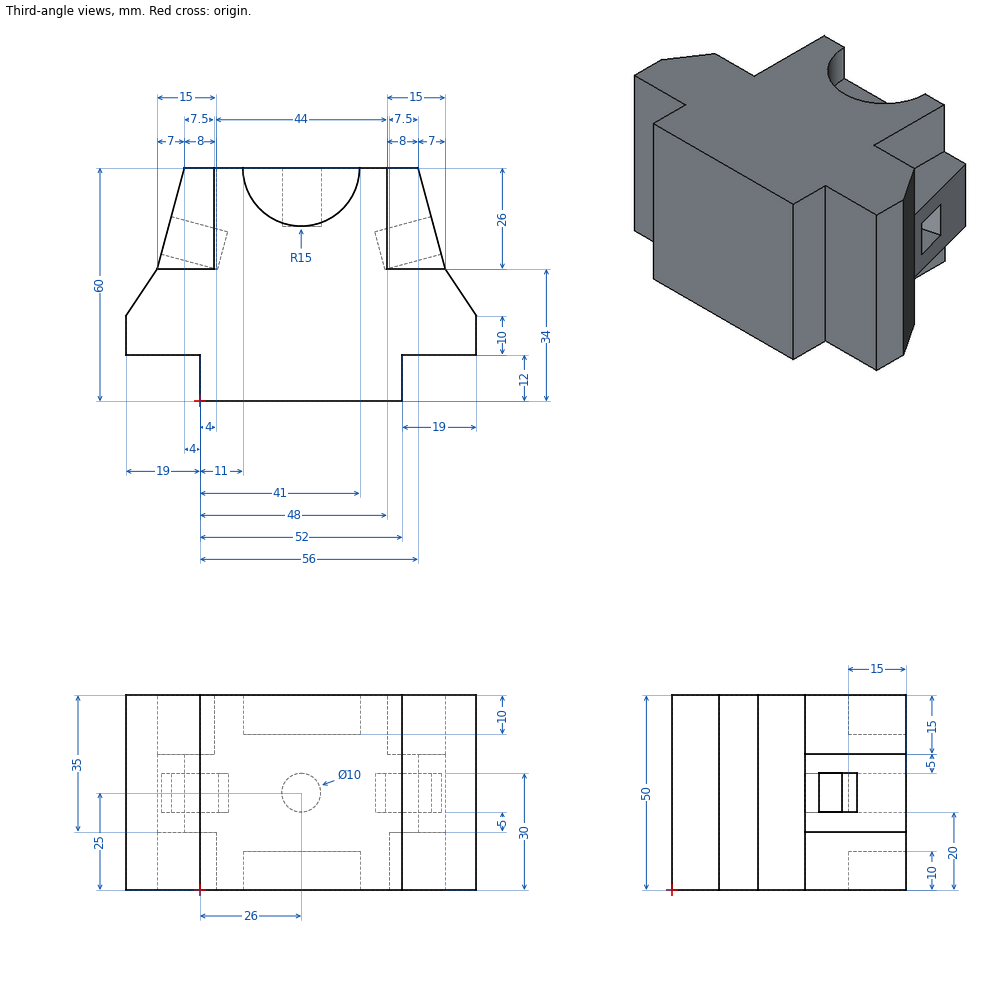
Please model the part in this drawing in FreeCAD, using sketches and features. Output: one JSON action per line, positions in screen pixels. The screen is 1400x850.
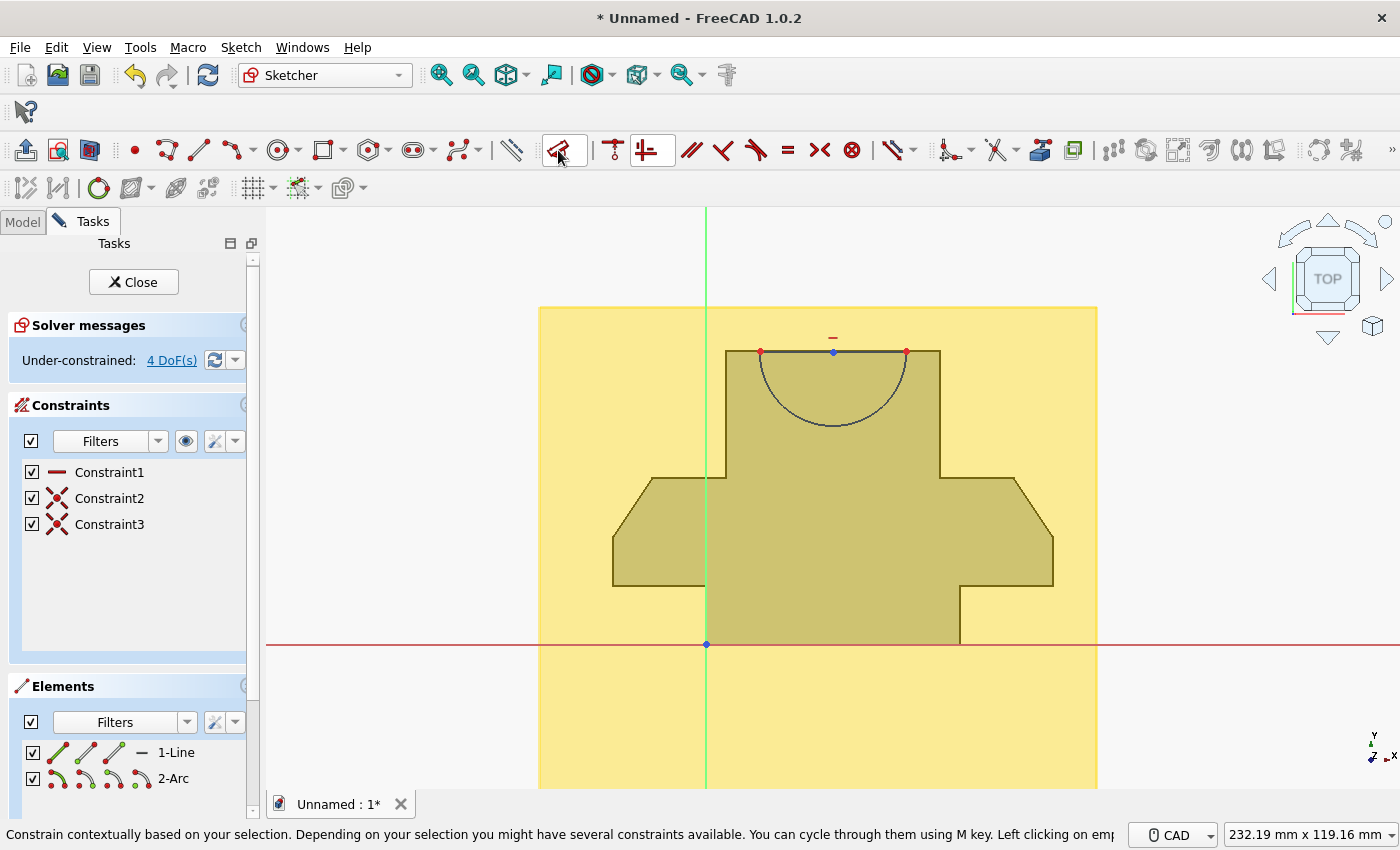
{"action": "left_click", "coordinate": [790, 412]}
{"action": "left_click", "coordinate": [771, 438]}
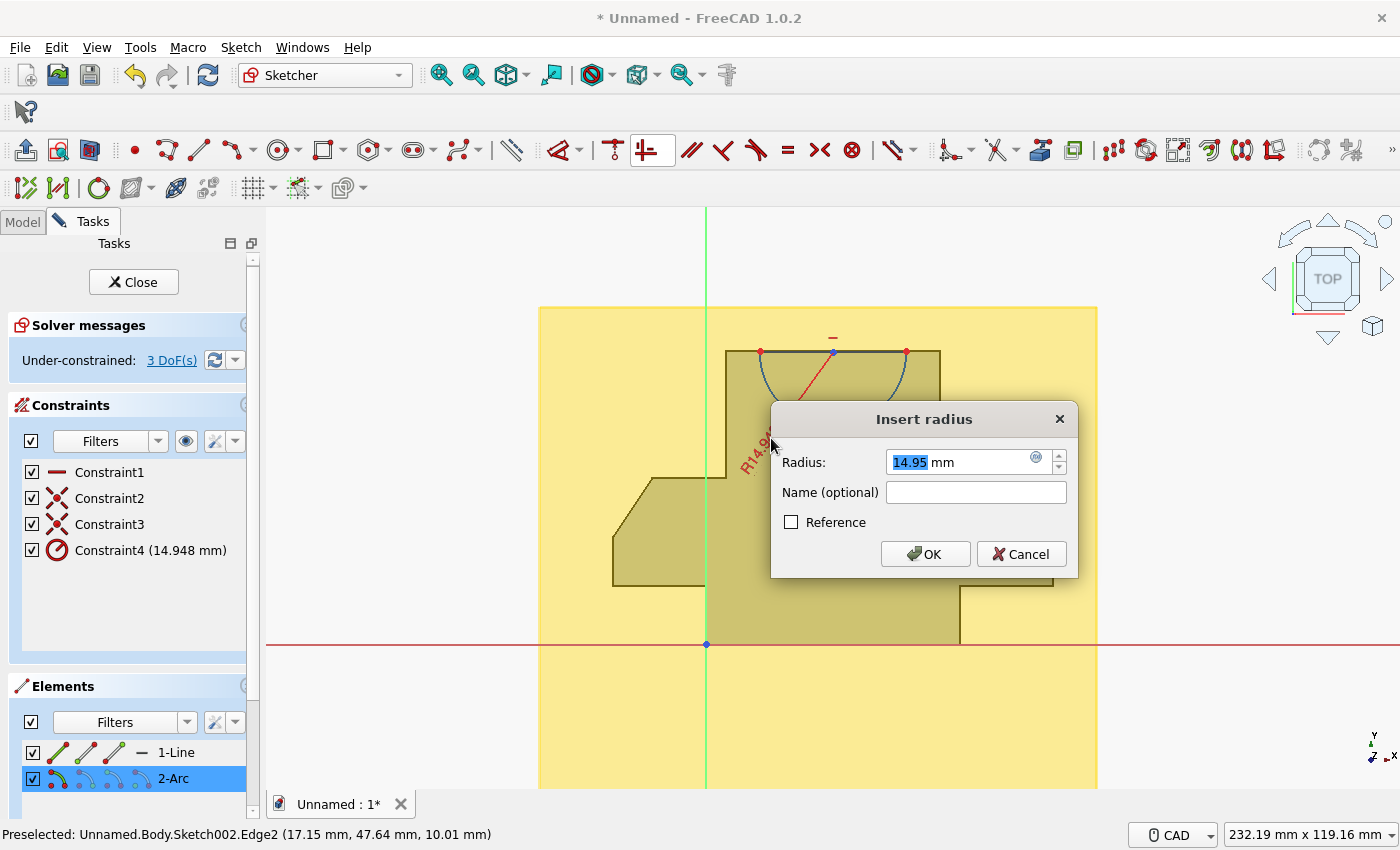
{"action": "type", "text": "15"}
{"action": "key", "text": "Return"}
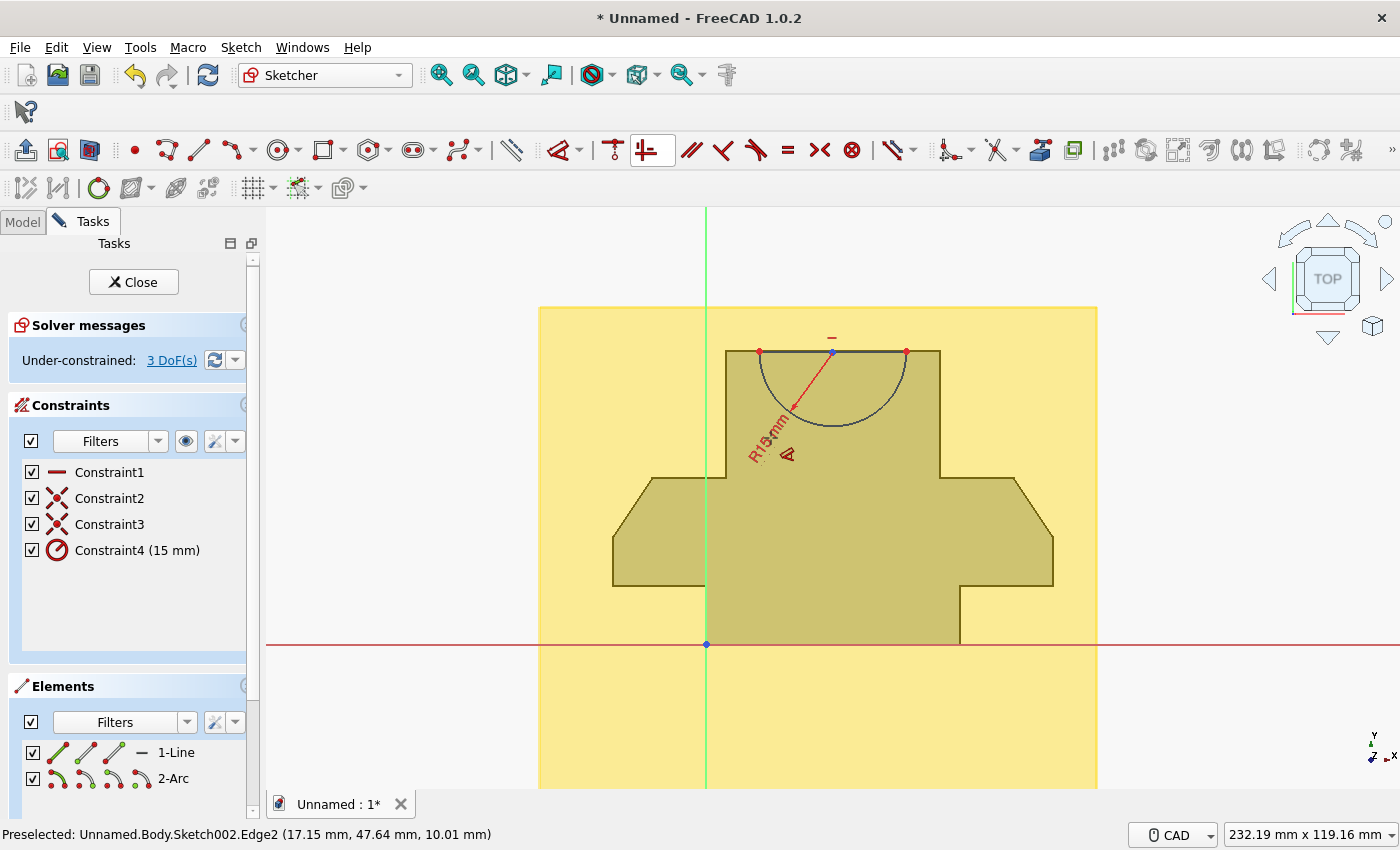
{"action": "left_click", "coordinate": [760, 352]}
{"action": "left_click", "coordinate": [733, 679]}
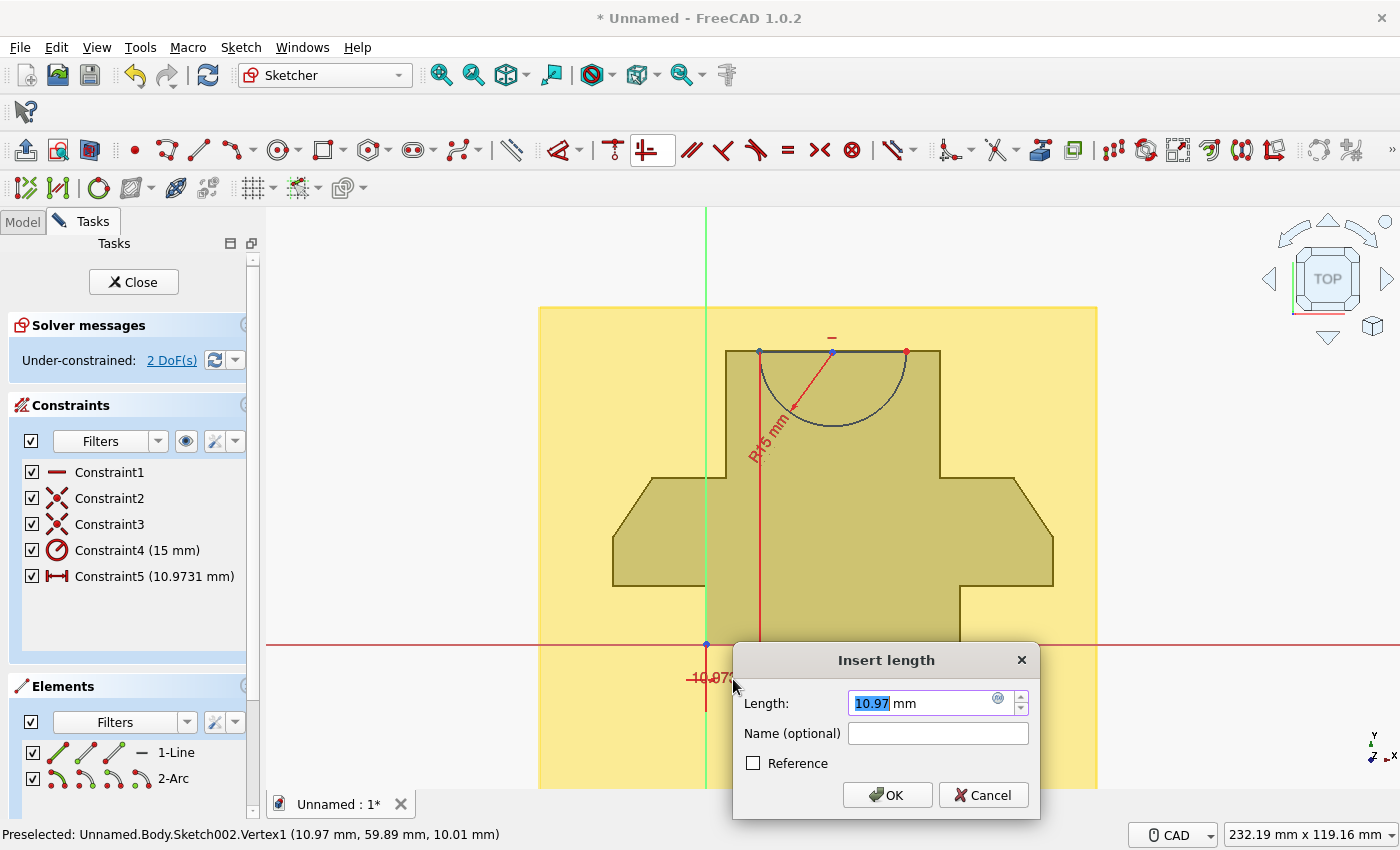
{"action": "type", "text": "11"}
{"action": "key", "text": "Return"}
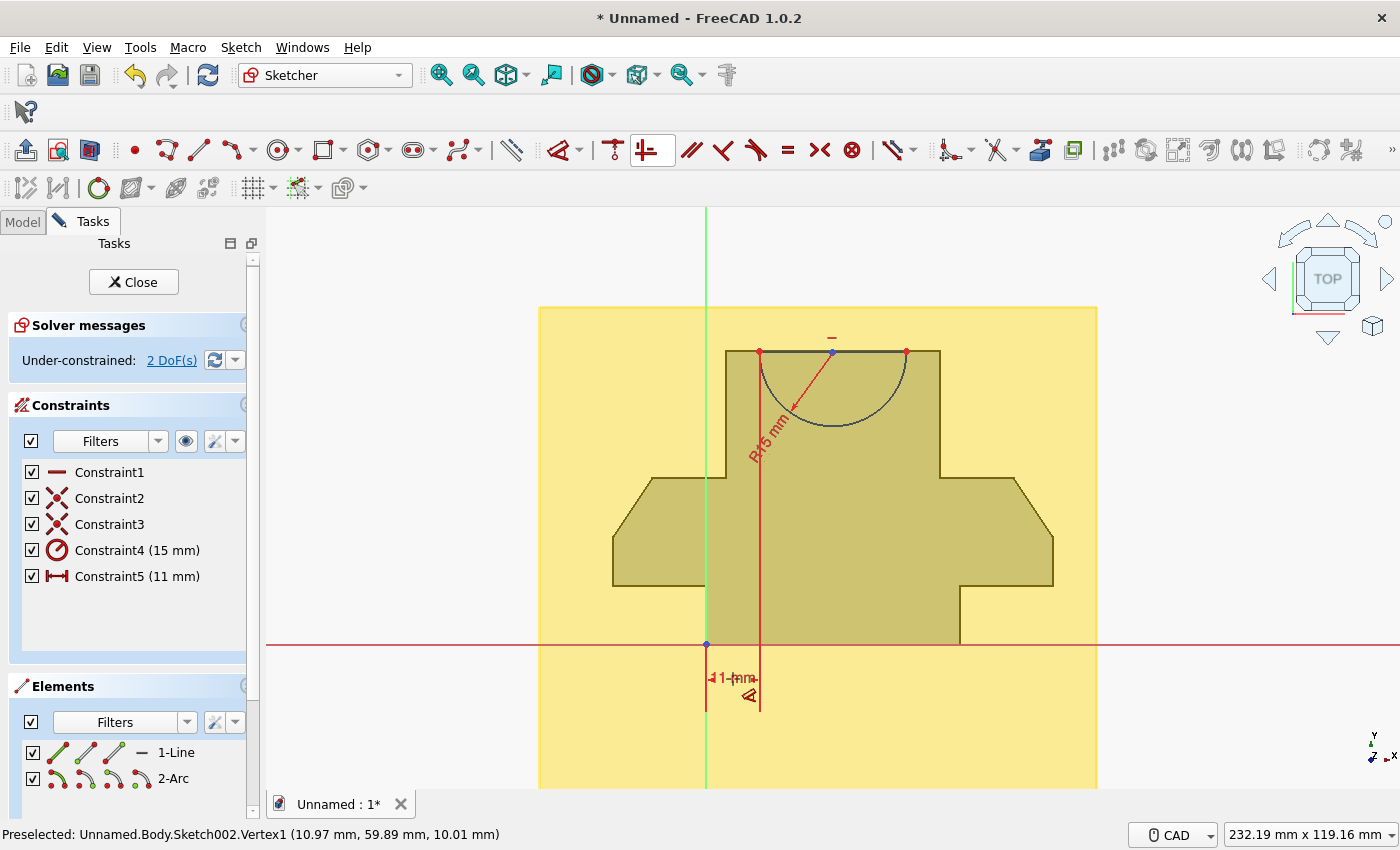
{"action": "left_click", "coordinate": [760, 352]}
{"action": "left_click", "coordinate": [672, 498]}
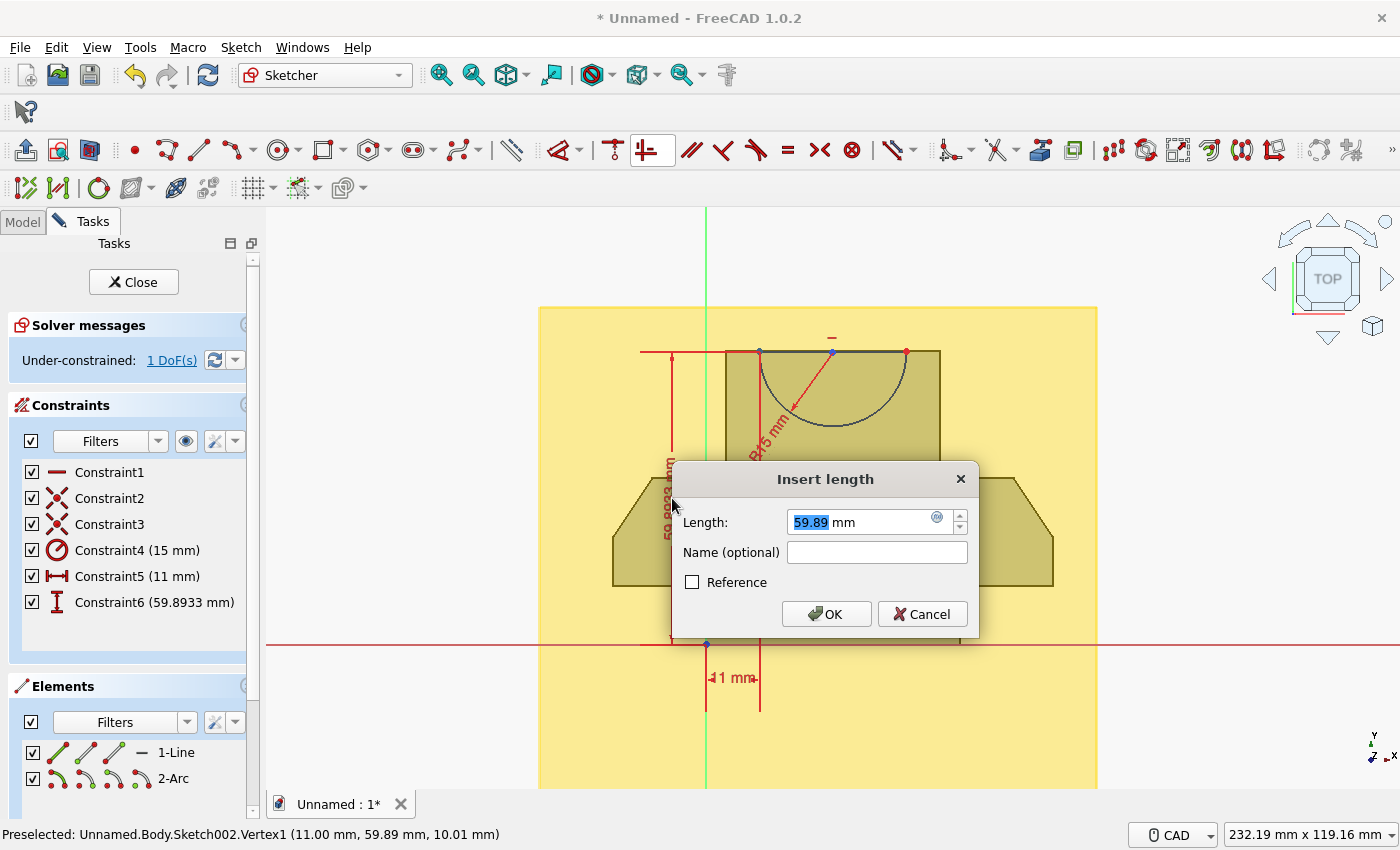
{"action": "type", "text": "60"}
{"action": "key", "text": "Return"}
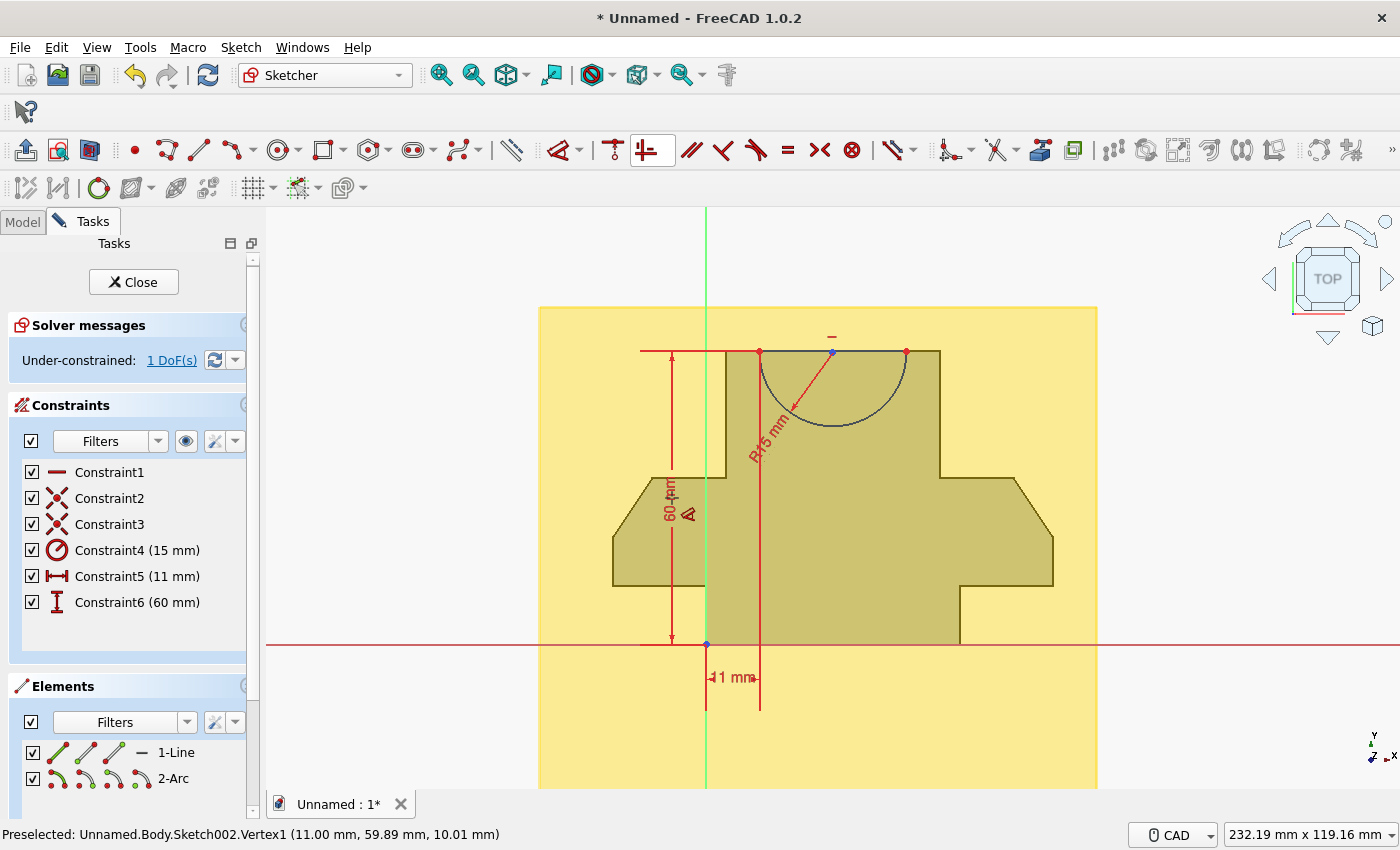
{"action": "left_click", "coordinate": [833, 353]}
{"action": "left_click", "coordinate": [672, 432]}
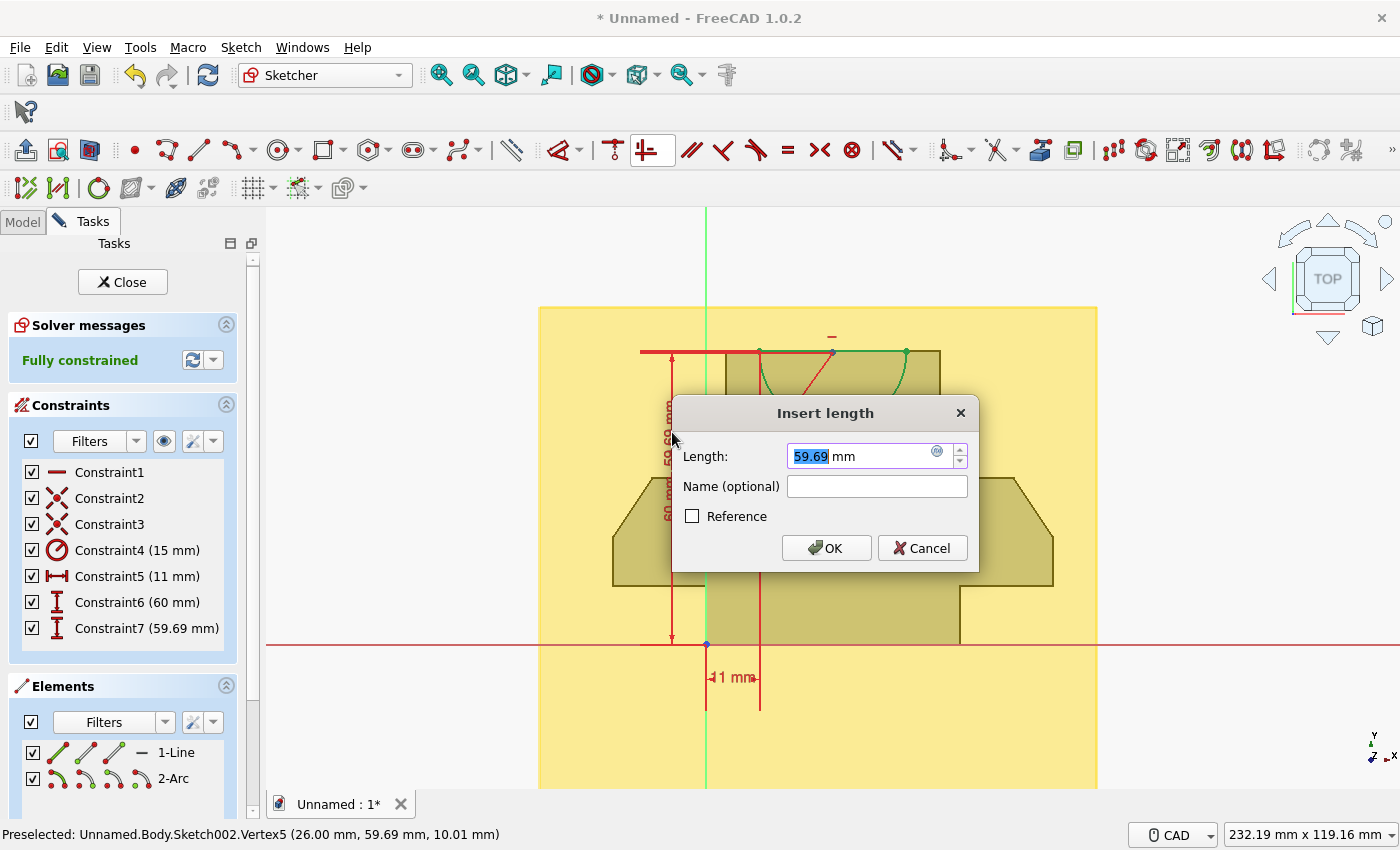
{"action": "type", "text": "60"}
{"action": "key", "text": "Return"}
{"action": "key", "text": "Escape"}